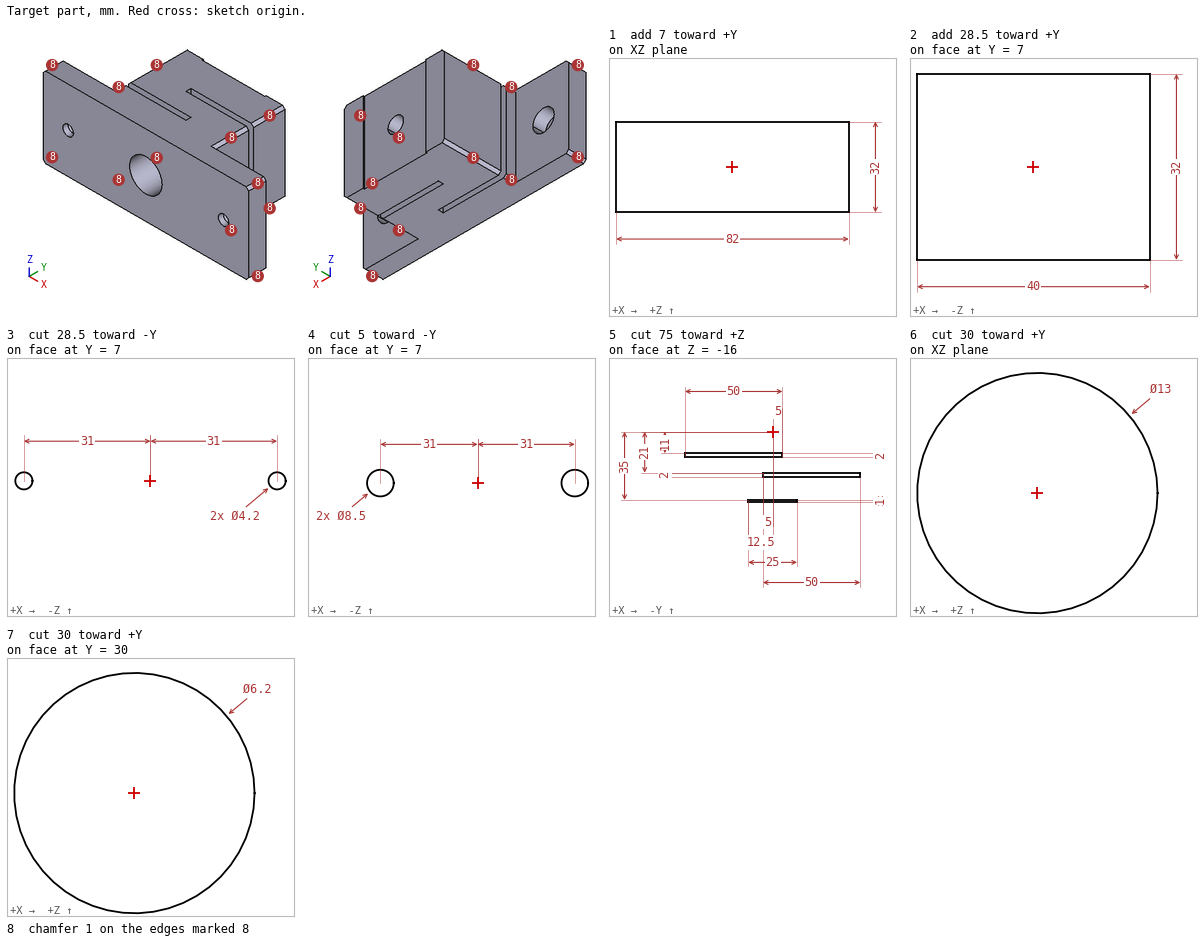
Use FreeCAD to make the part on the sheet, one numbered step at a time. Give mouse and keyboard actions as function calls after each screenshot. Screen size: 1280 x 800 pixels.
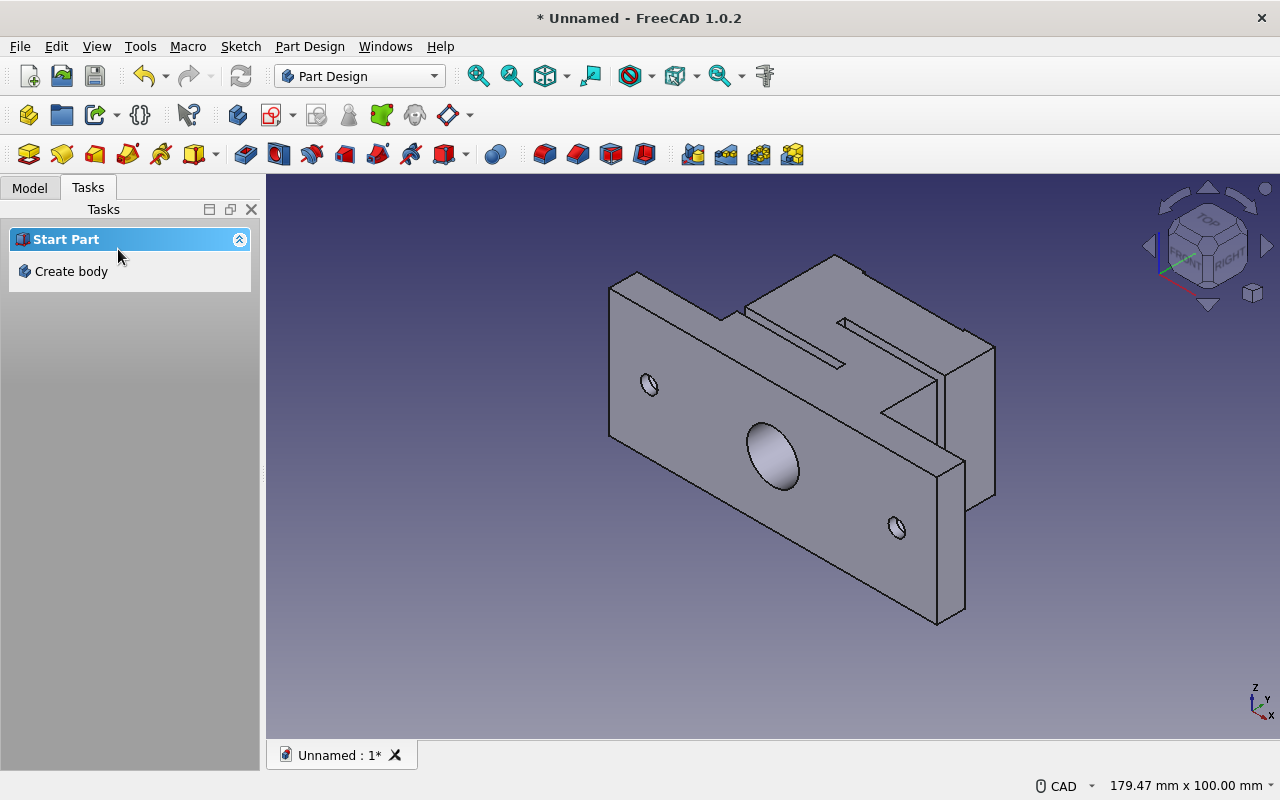
key(1)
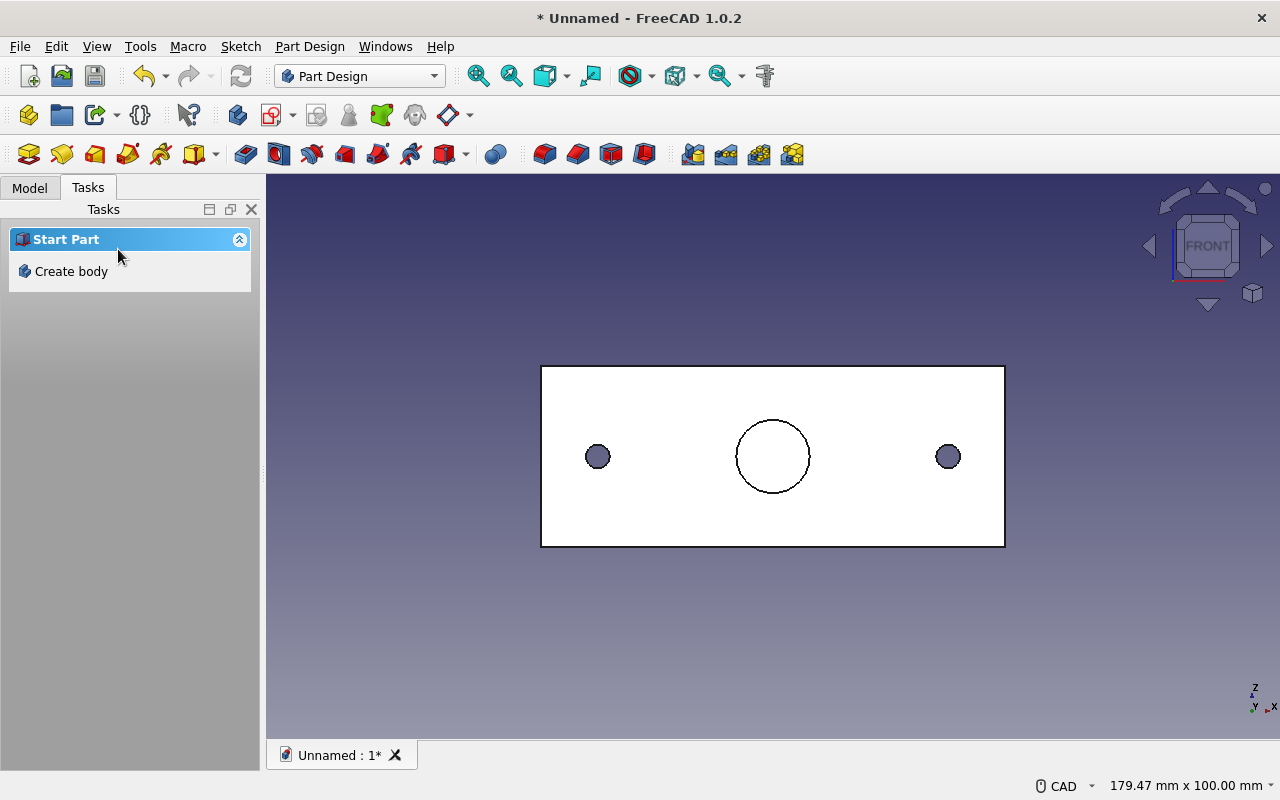
click(773, 456)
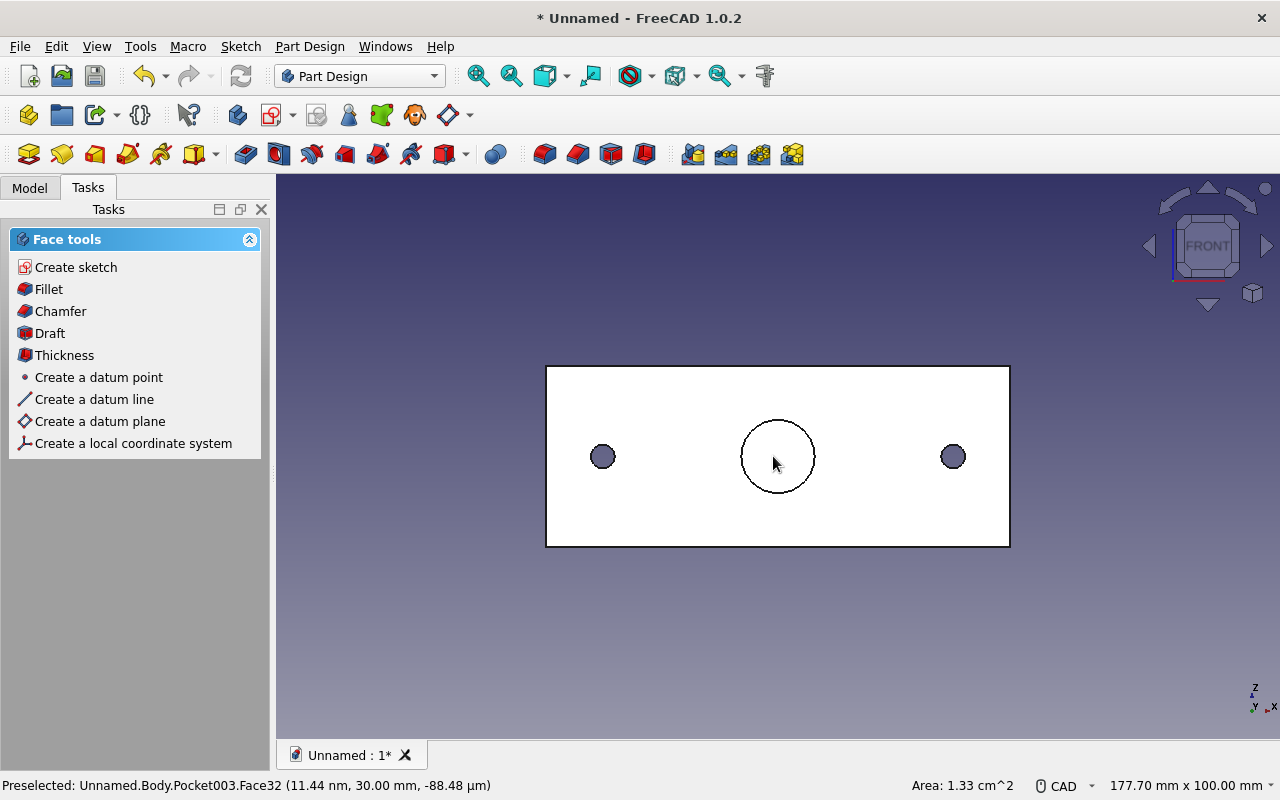
click(270, 116)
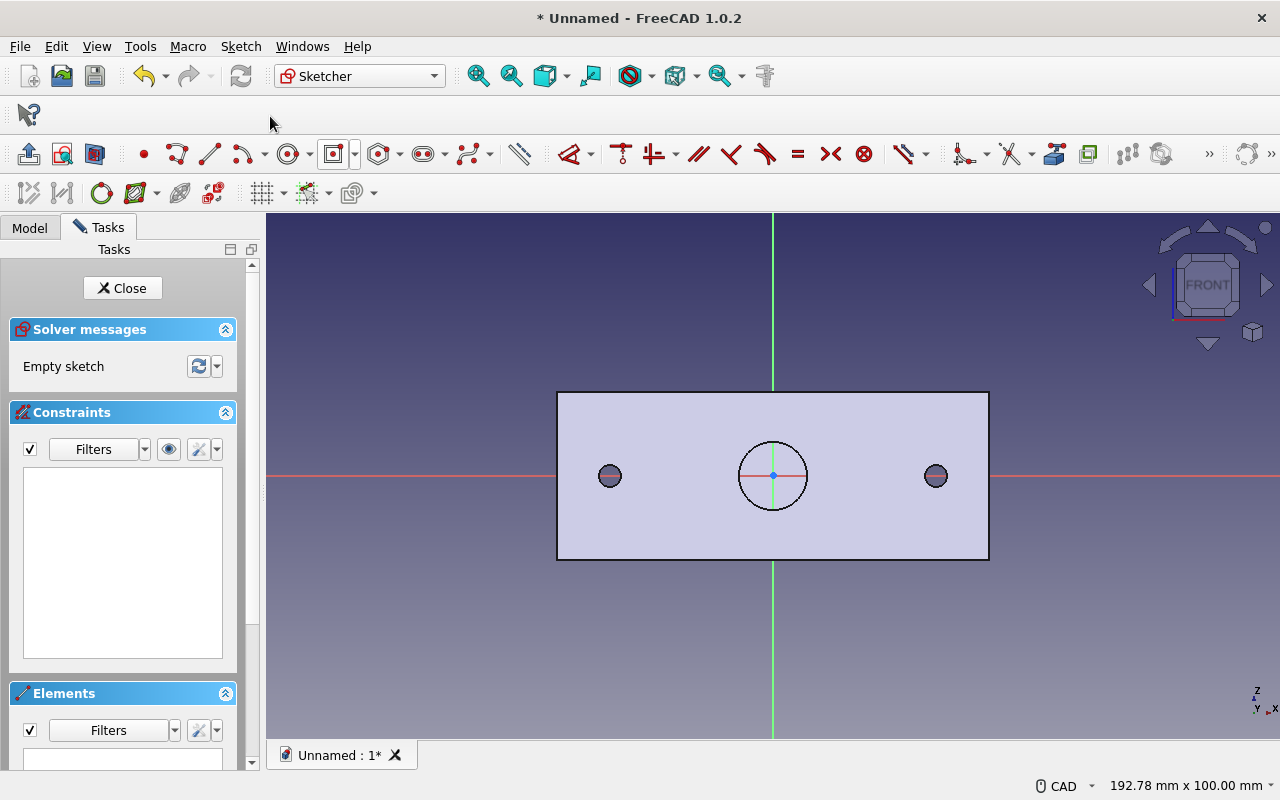
click(95, 154)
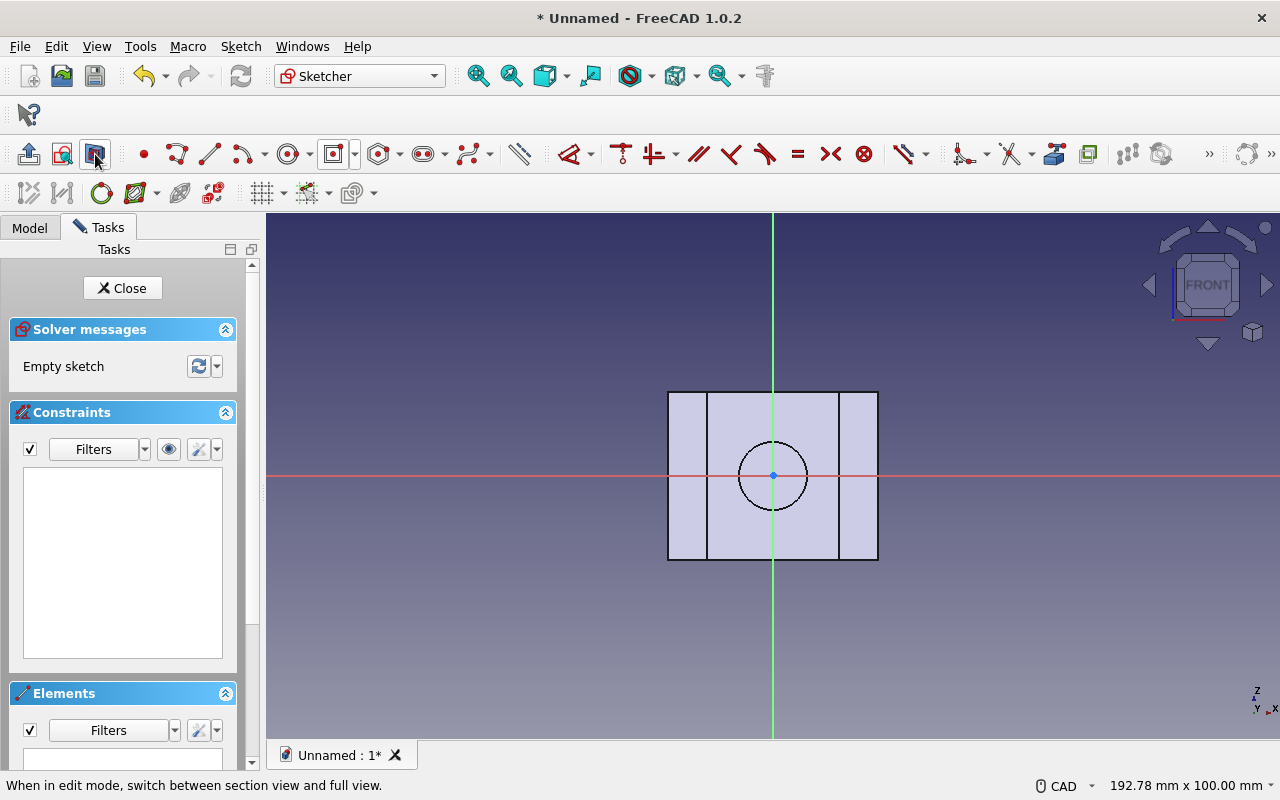
scroll(780, 476, up, 12)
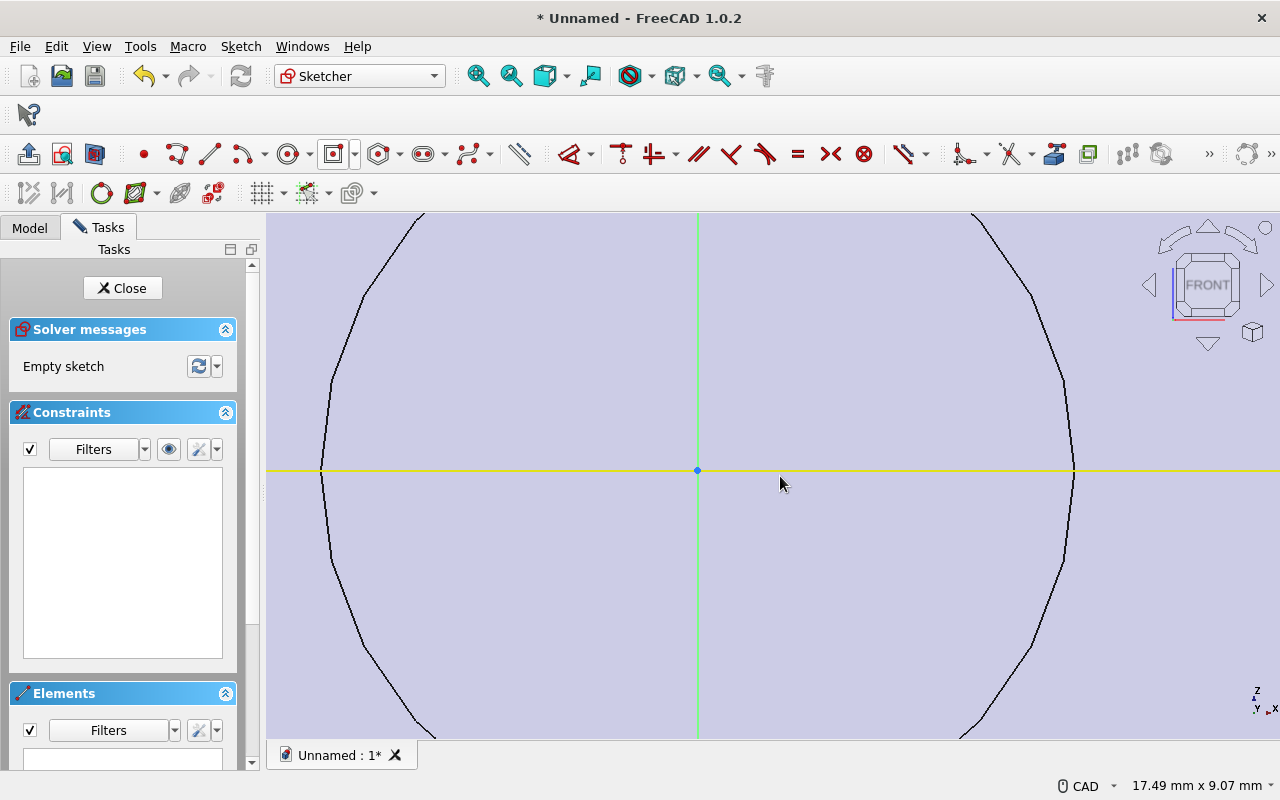
click(288, 154)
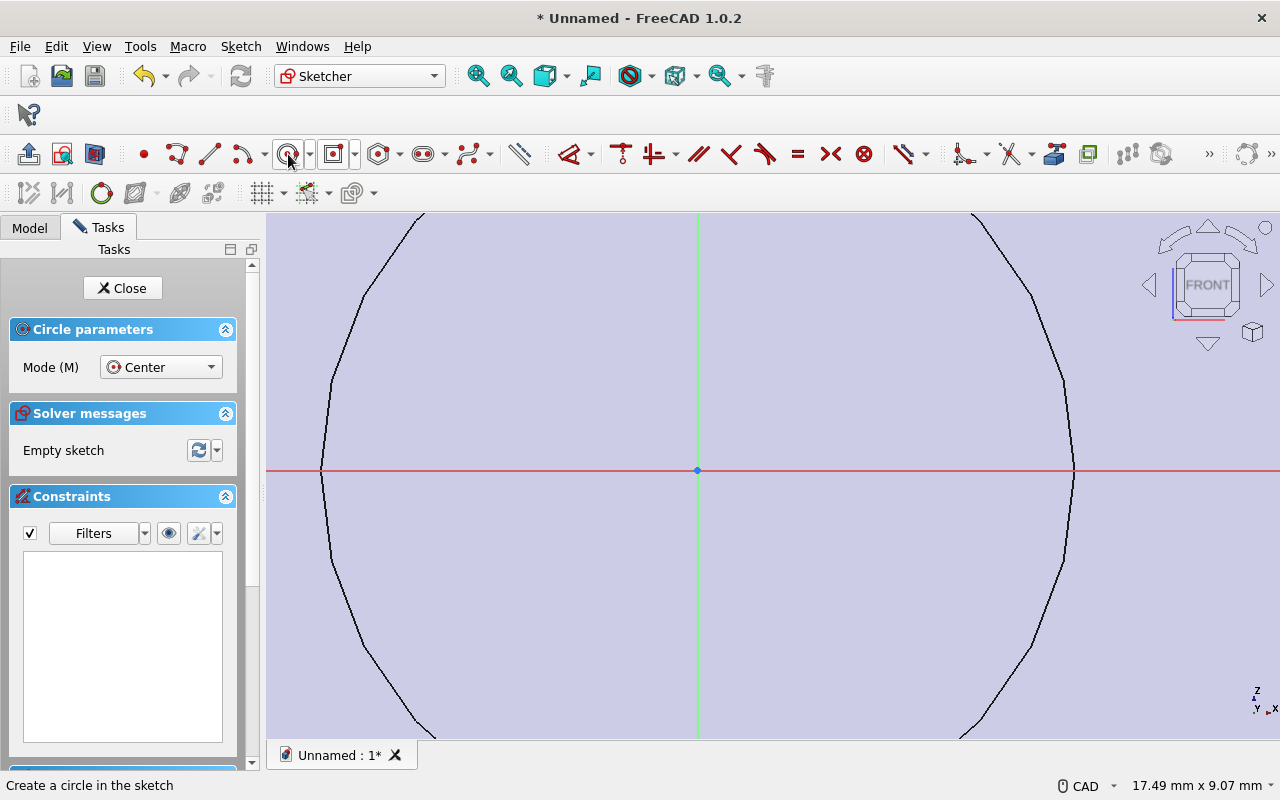
click(698, 471)
move(825, 344)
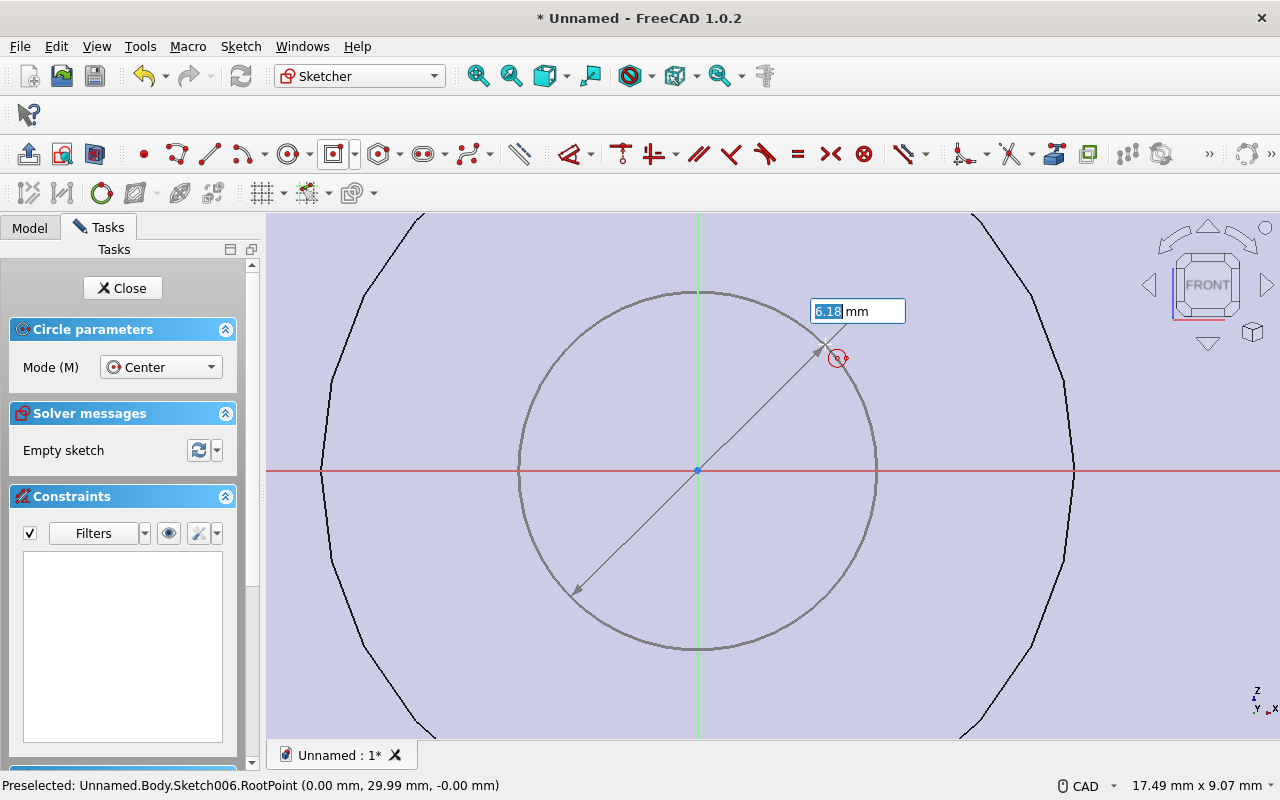
text(6.2)
key(Return)
key(Escape)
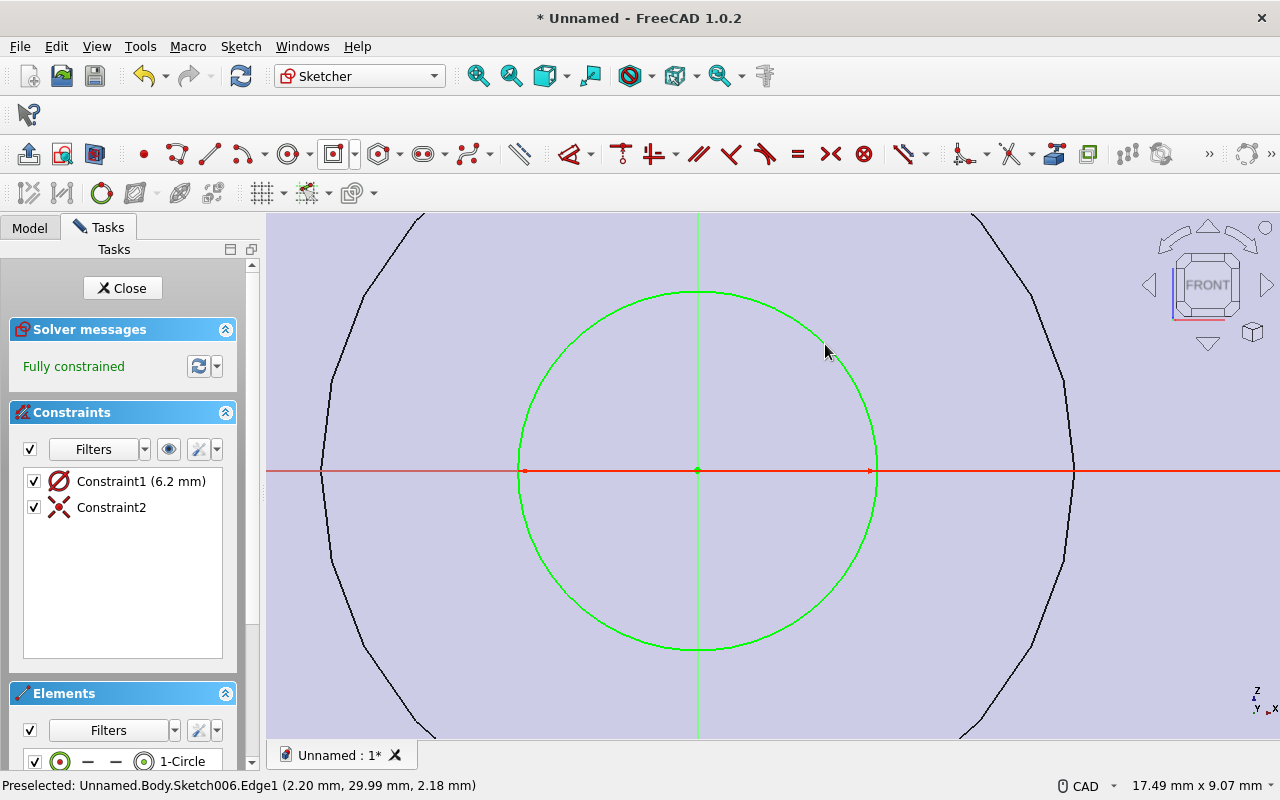
click(123, 288)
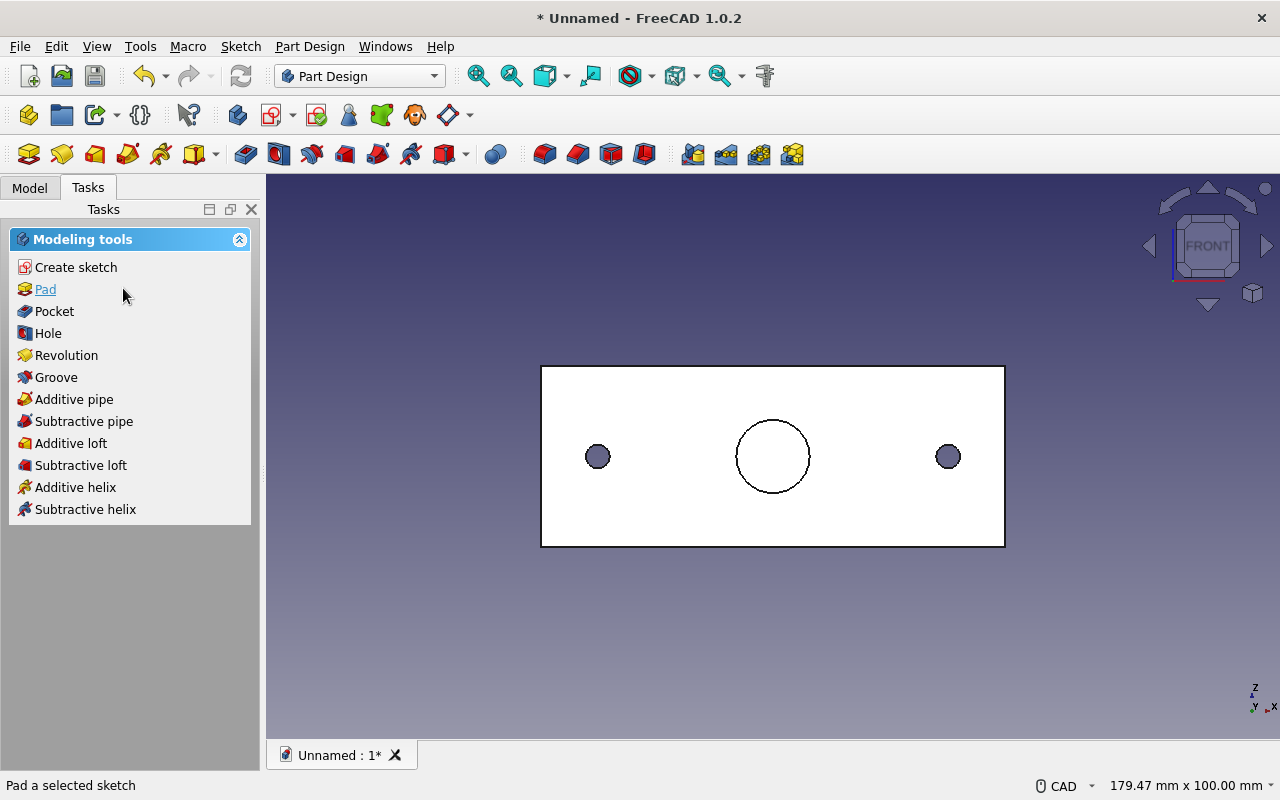
click(246, 154)